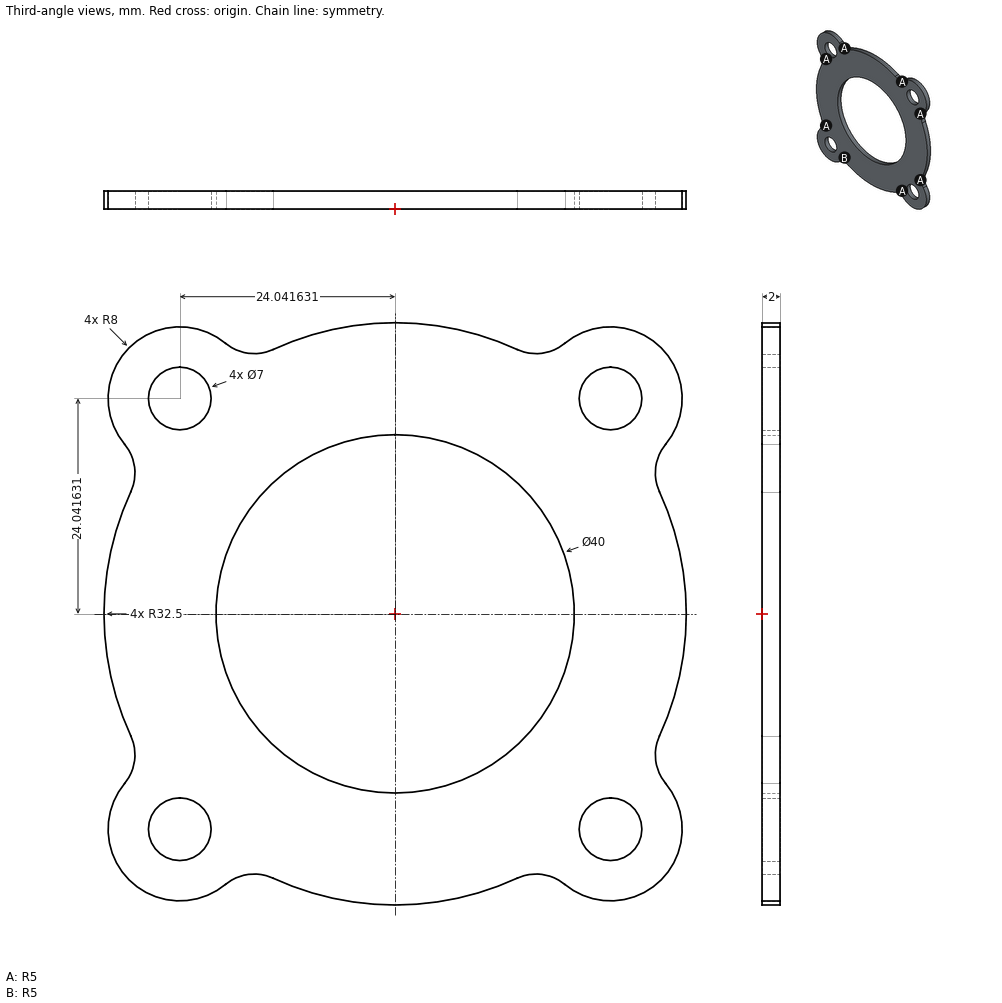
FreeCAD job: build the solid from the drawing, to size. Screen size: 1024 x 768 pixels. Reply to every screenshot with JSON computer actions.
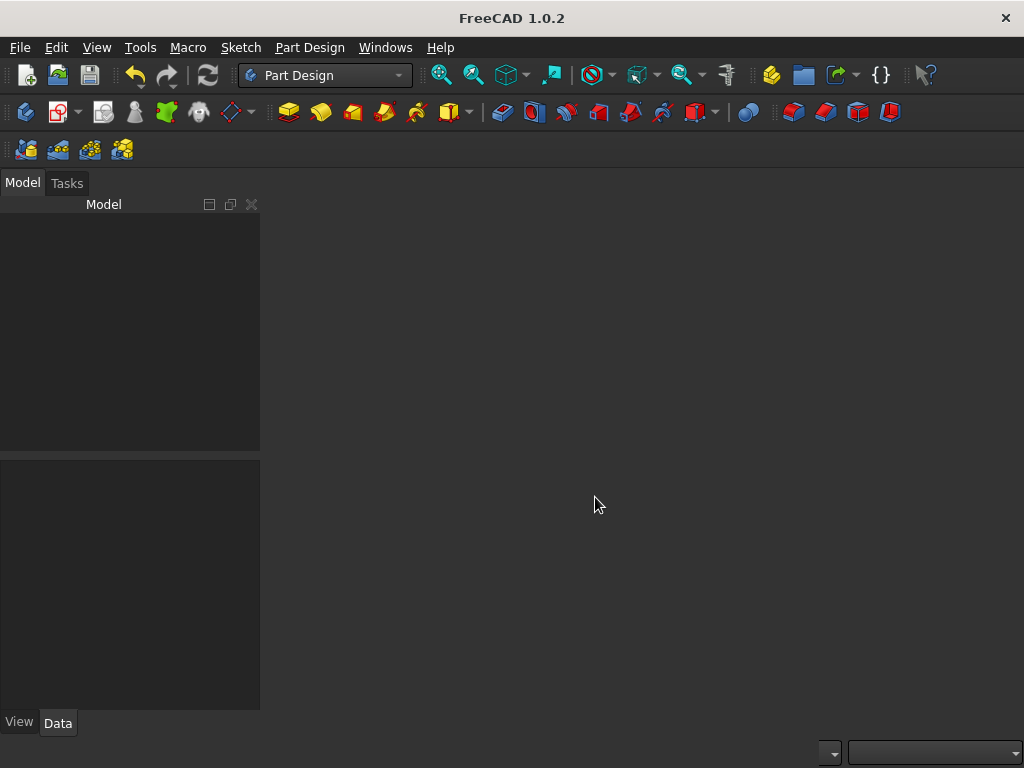
{"action": "left_click", "coordinate": [26, 76]}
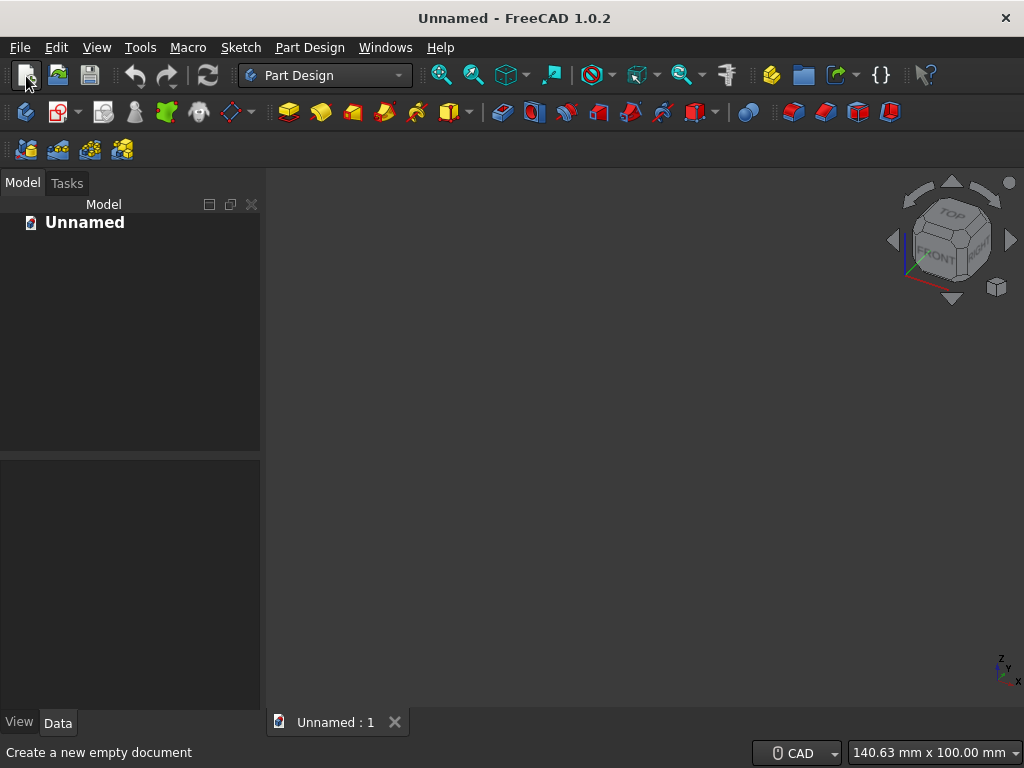
{"action": "left_click", "coordinate": [58, 112]}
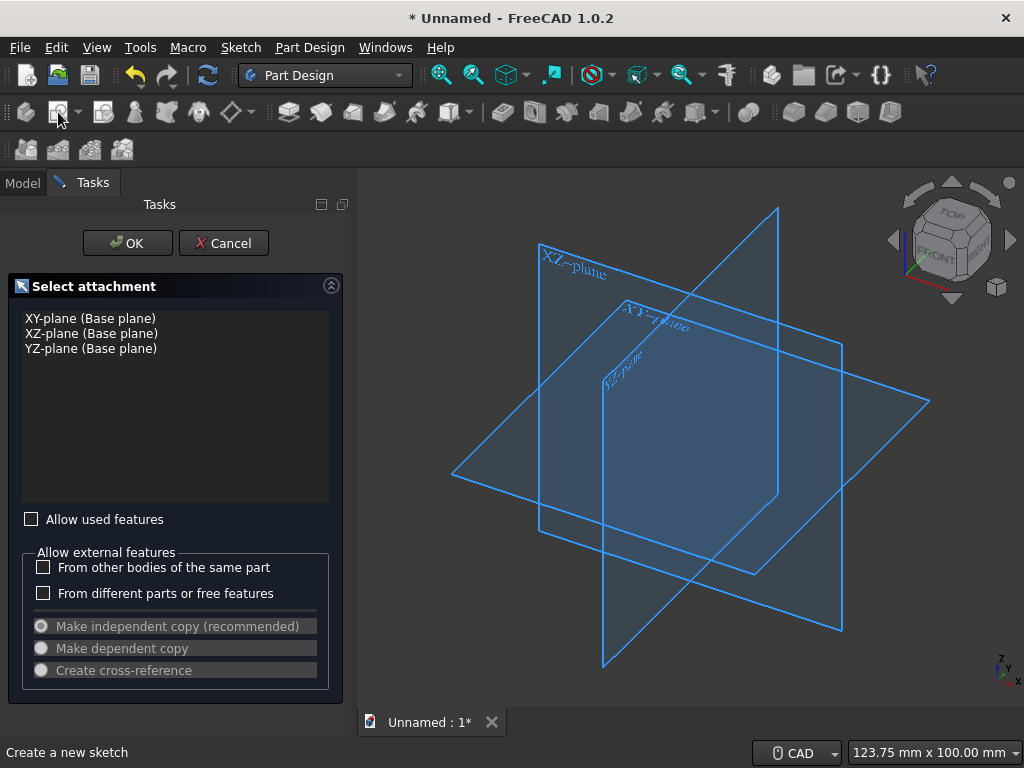
{"action": "left_click", "coordinate": [82, 334]}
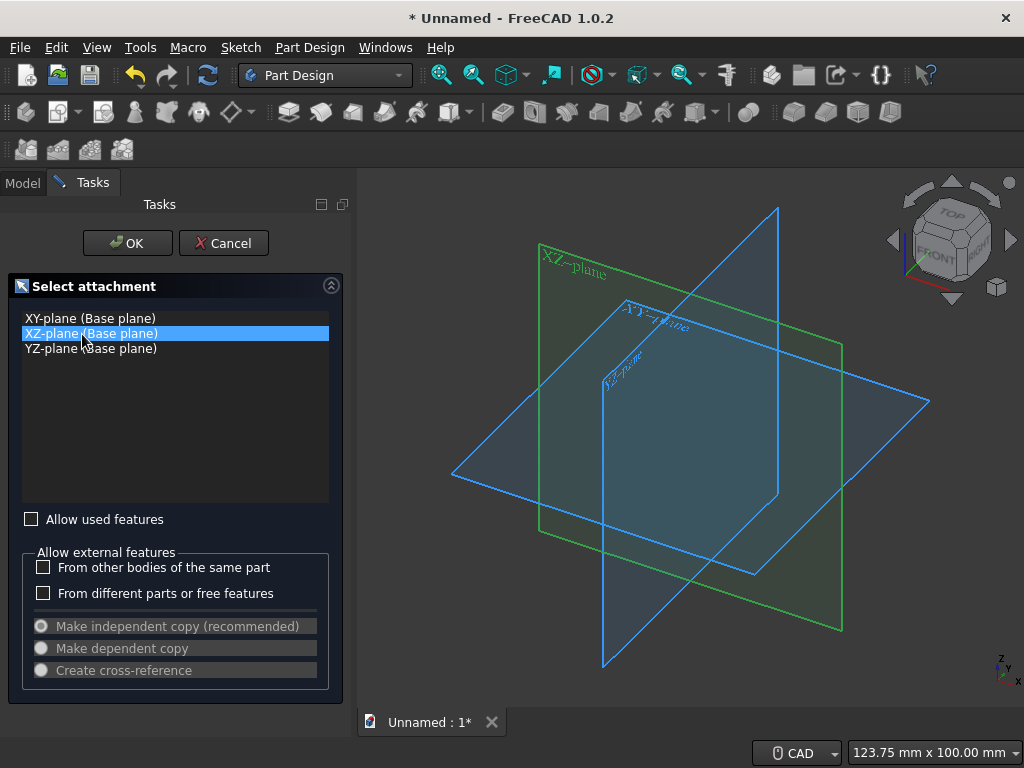
{"action": "left_click", "coordinate": [128, 243]}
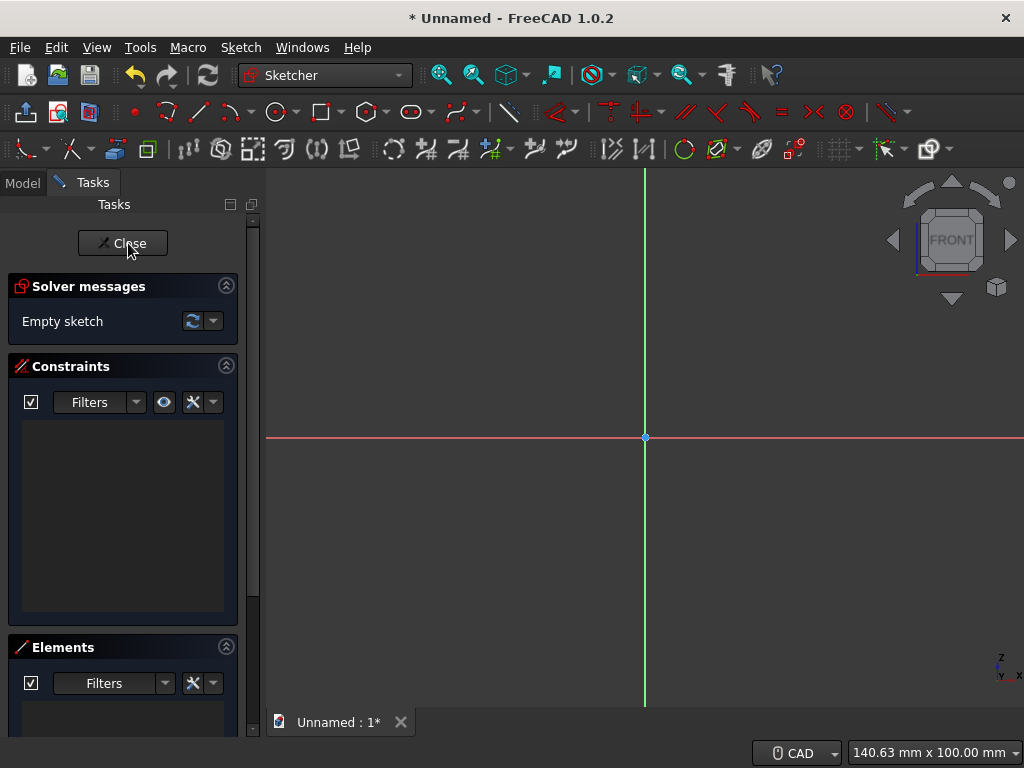
{"action": "key", "text": "g 3 a"}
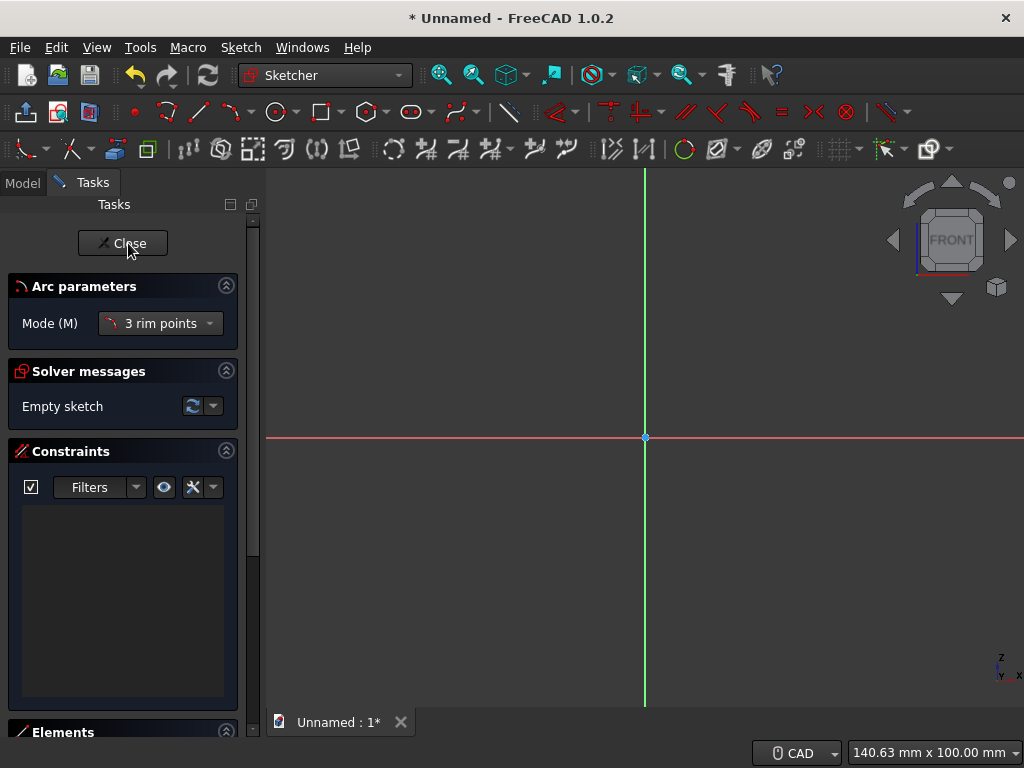
{"action": "left_click", "coordinate": [496, 529]}
{"action": "left_click", "coordinate": [496, 346]}
{"action": "left_click", "coordinate": [471, 418]}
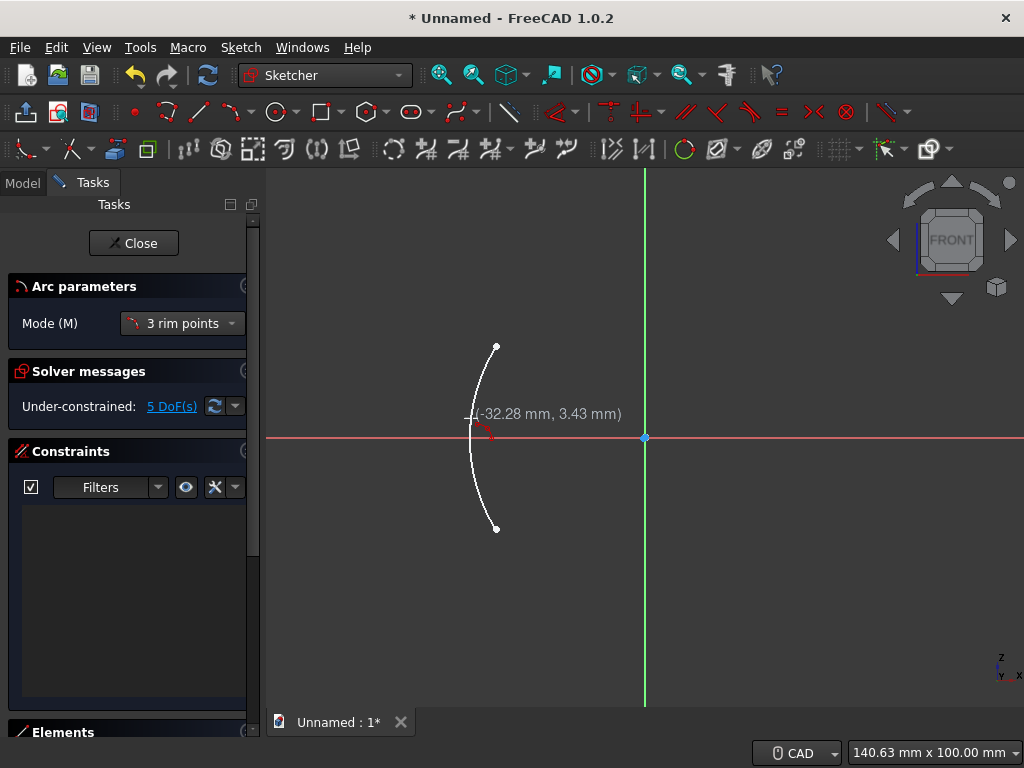
{"action": "left_click", "coordinate": [496, 347]}
{"action": "left_click", "coordinate": [554, 288]}
{"action": "left_click", "coordinate": [485, 277]}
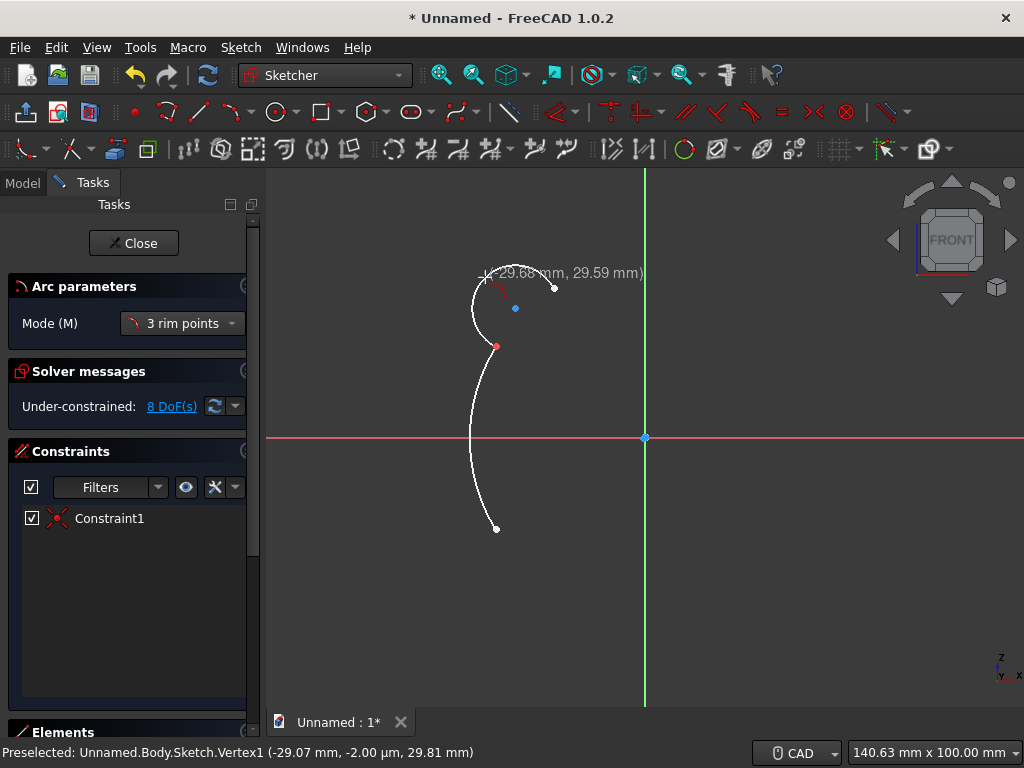
{"action": "left_click", "coordinate": [554, 289]}
{"action": "left_click", "coordinate": [736, 288]}
{"action": "left_click", "coordinate": [664, 263]}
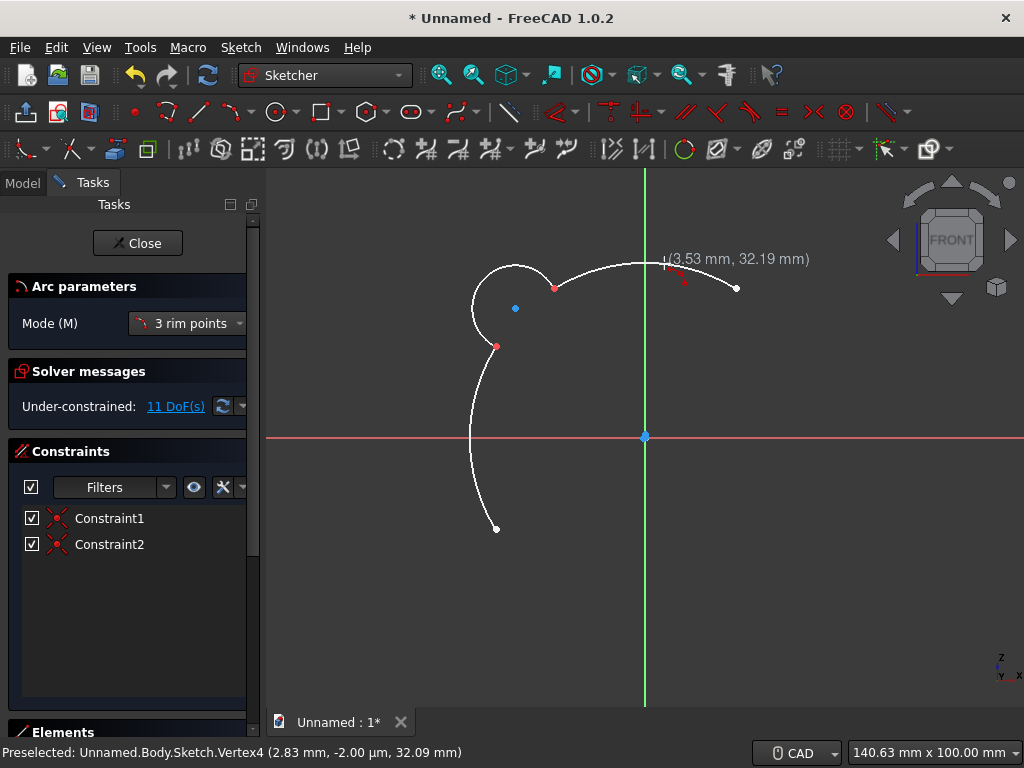
{"action": "left_click", "coordinate": [736, 289]}
{"action": "left_click", "coordinate": [794, 346]}
{"action": "left_click", "coordinate": [805, 277]}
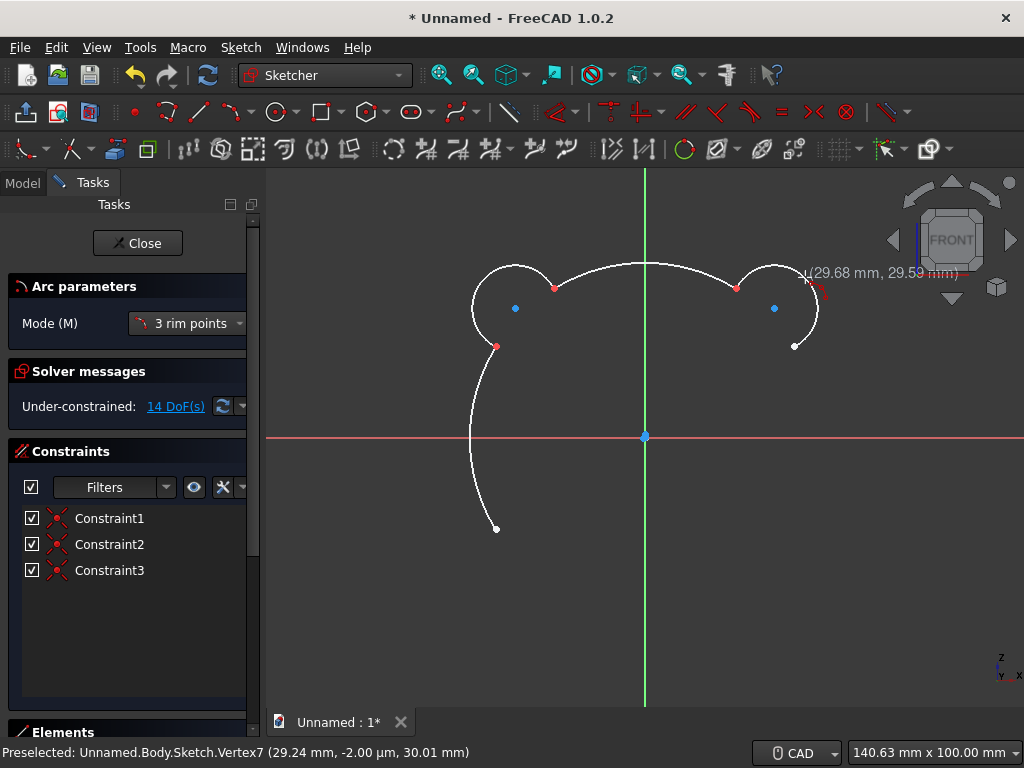
{"action": "left_click", "coordinate": [794, 347]}
{"action": "left_click", "coordinate": [794, 529]}
{"action": "left_click", "coordinate": [819, 457]}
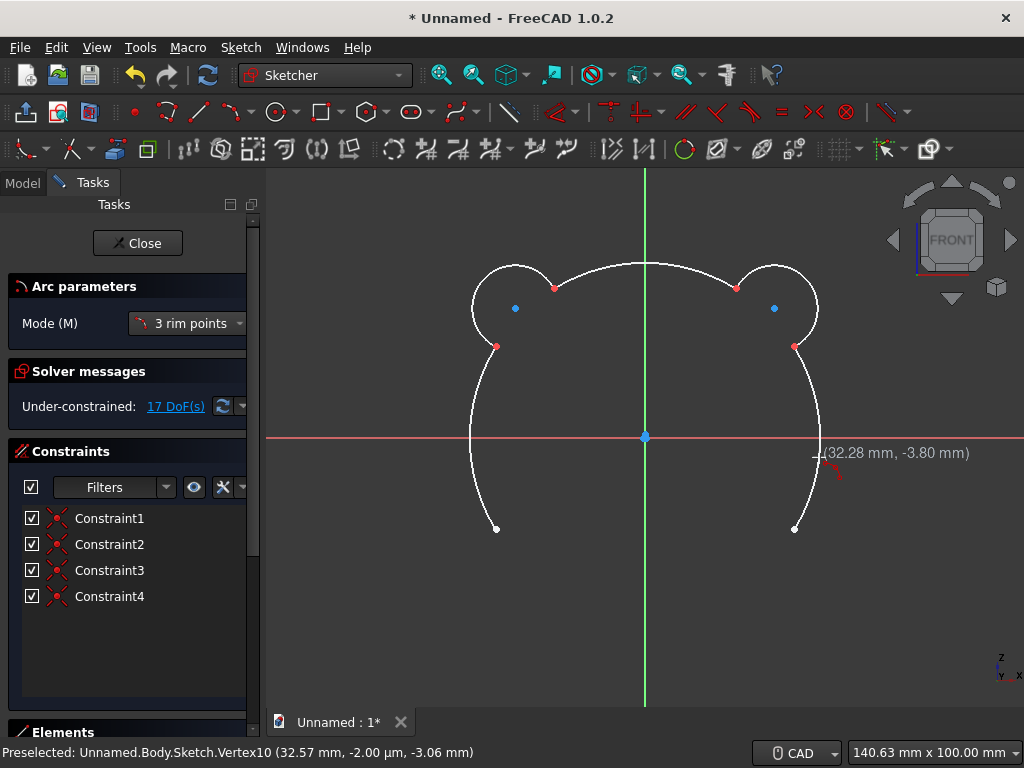
{"action": "left_click", "coordinate": [794, 530]}
{"action": "left_click", "coordinate": [736, 587]}
{"action": "left_click", "coordinate": [805, 598]}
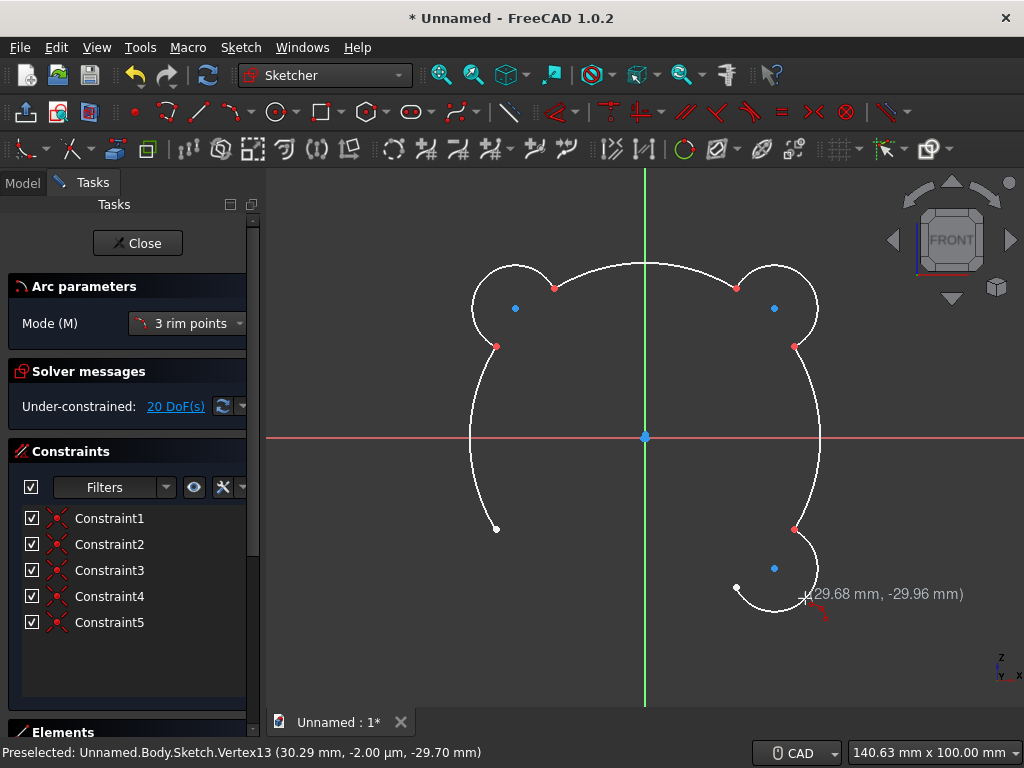
{"action": "left_click", "coordinate": [736, 588]}
{"action": "left_click", "coordinate": [554, 587]}
{"action": "left_click", "coordinate": [626, 612]}